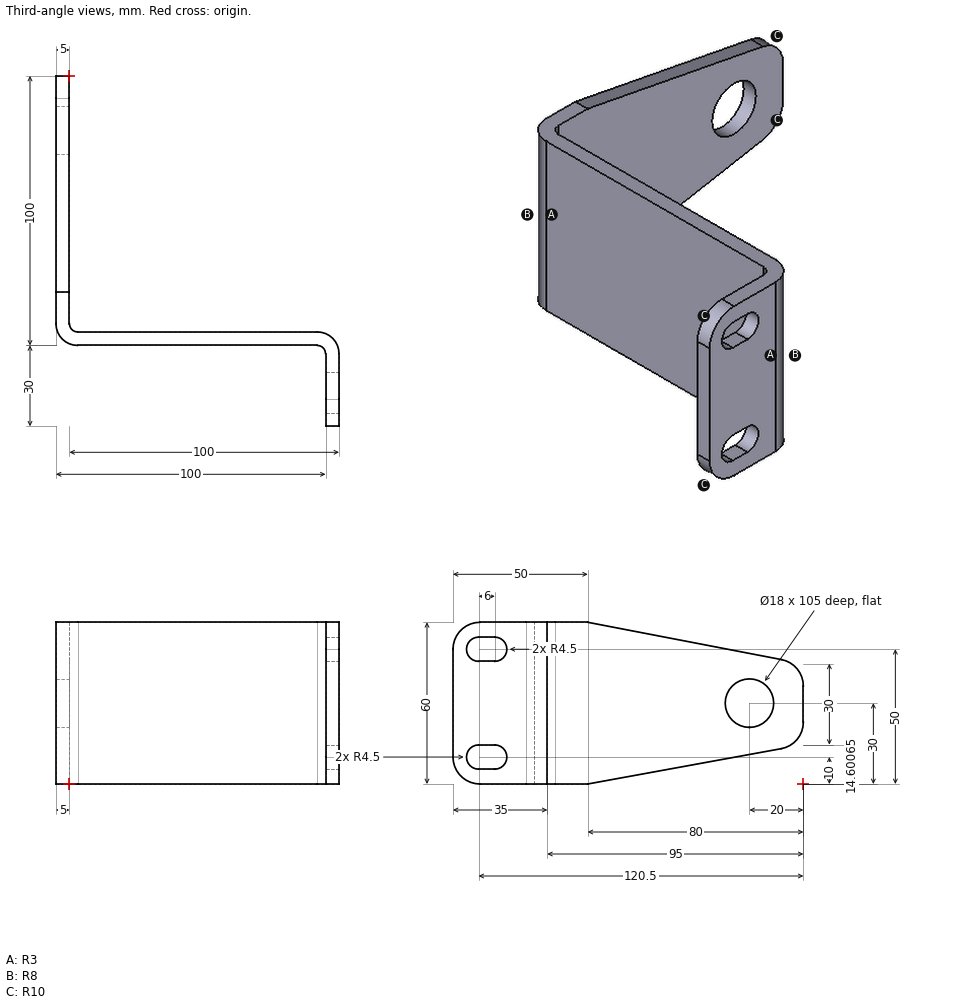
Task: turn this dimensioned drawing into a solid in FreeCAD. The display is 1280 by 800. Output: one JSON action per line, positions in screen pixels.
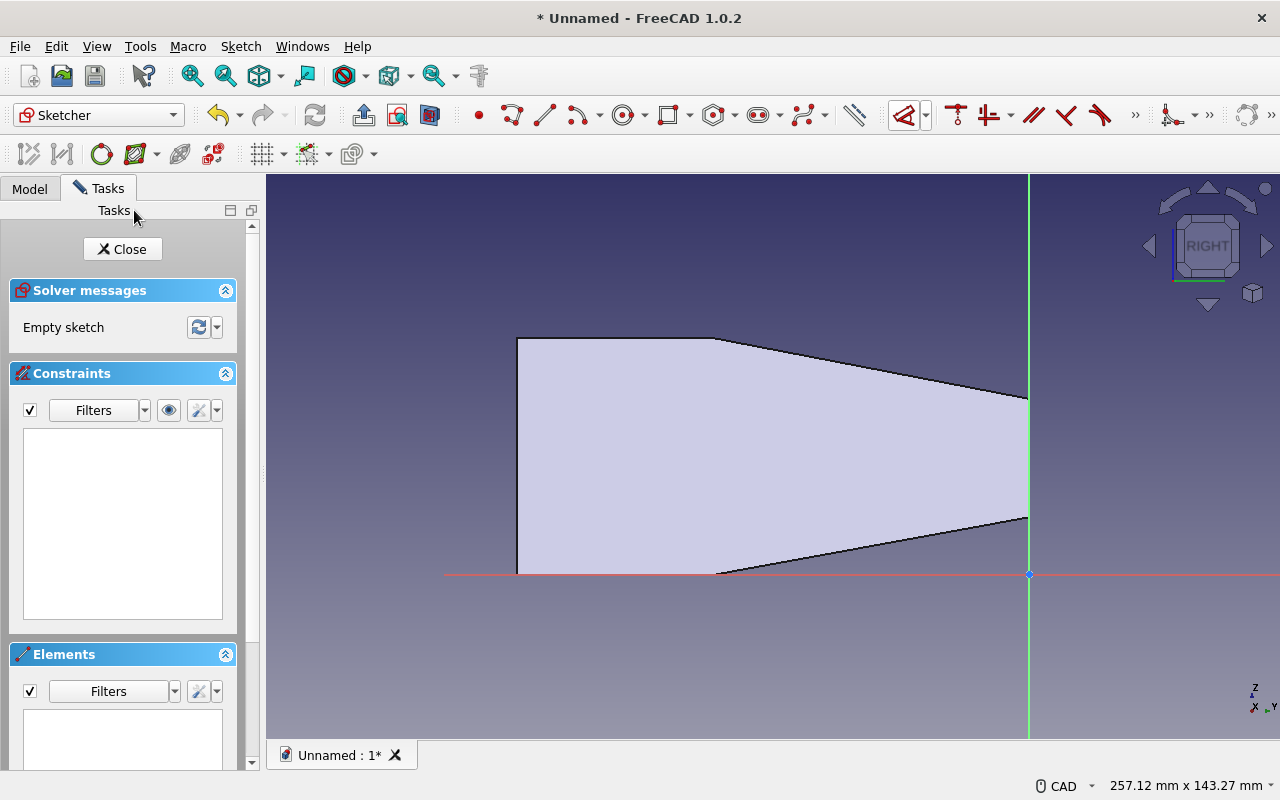
{"action": "left_click", "coordinate": [668, 116]}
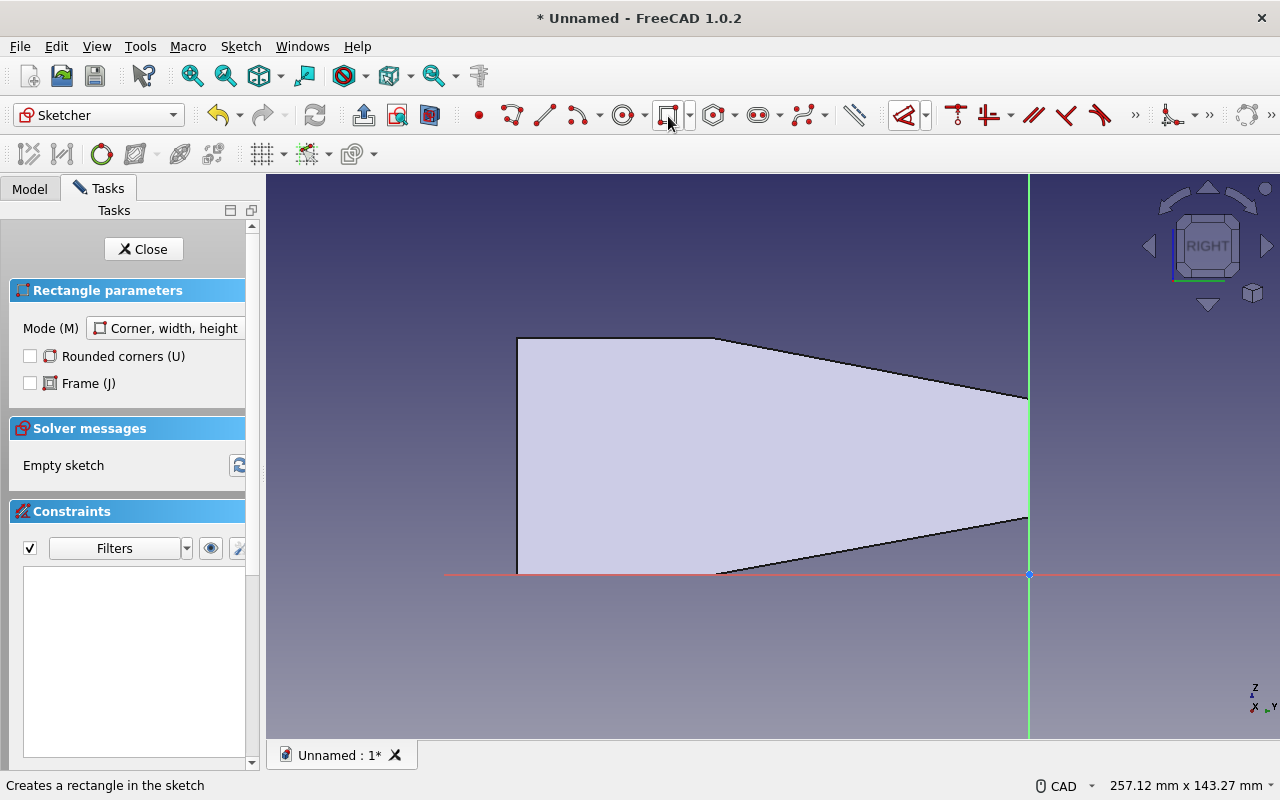
{"action": "left_click", "coordinate": [517, 338]}
{"action": "left_click", "coordinate": [655, 575]}
{"action": "key", "text": "Escape"}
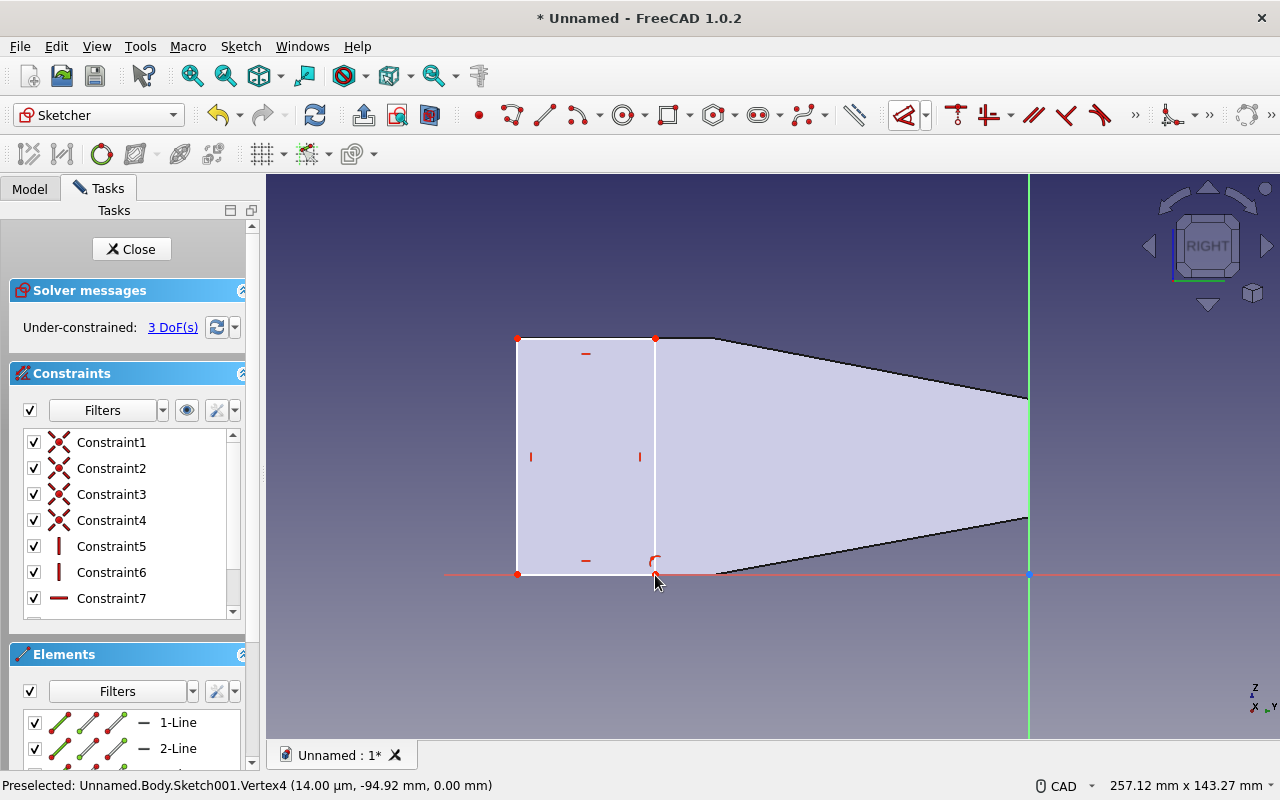
{"action": "left_click", "coordinate": [517, 410]}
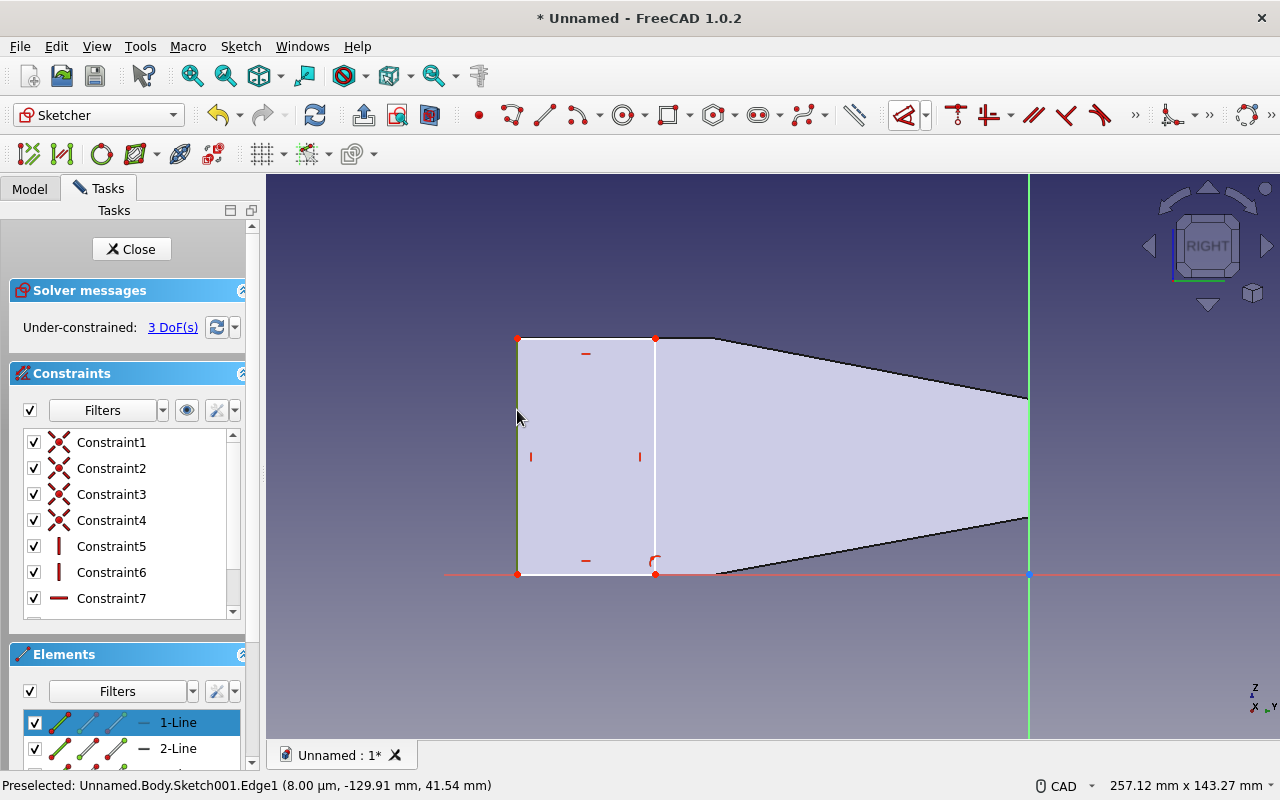
{"action": "key", "text": "i"}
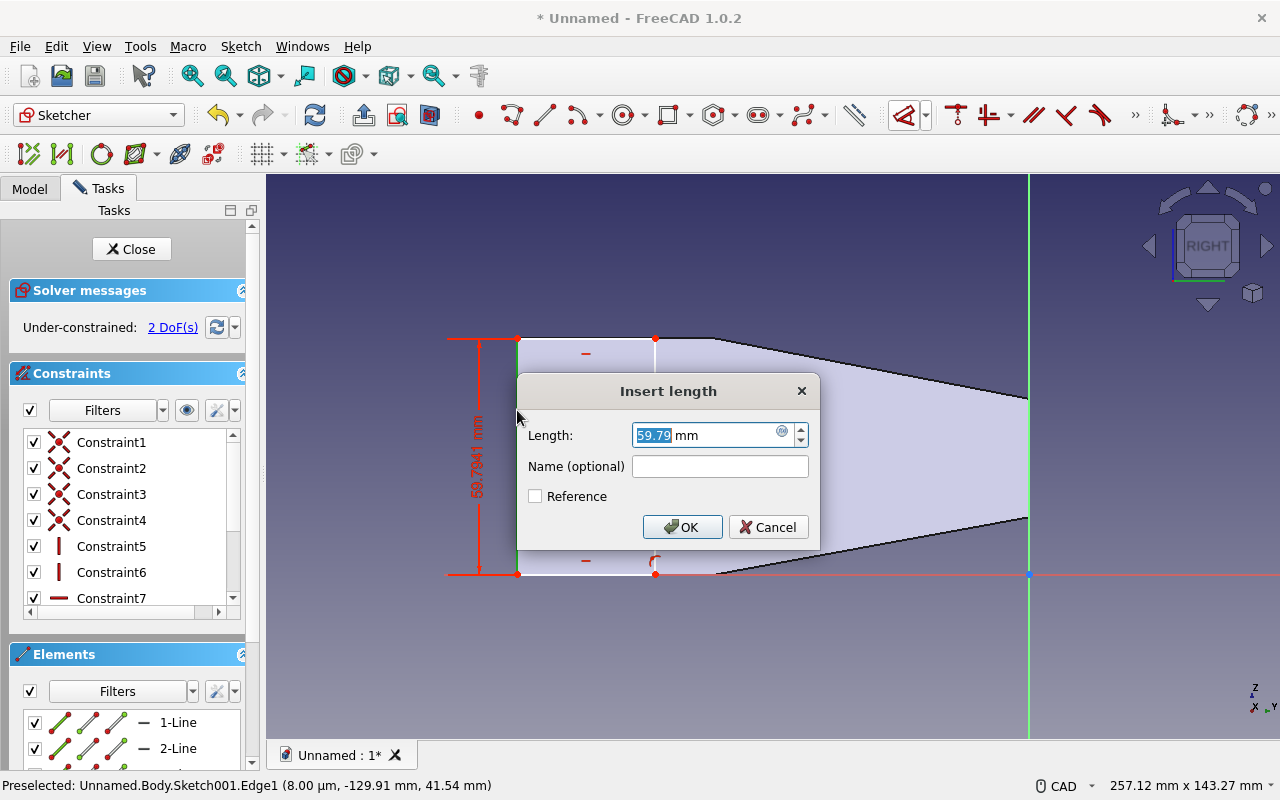
{"action": "type", "text": "60"}
{"action": "key", "text": "Return"}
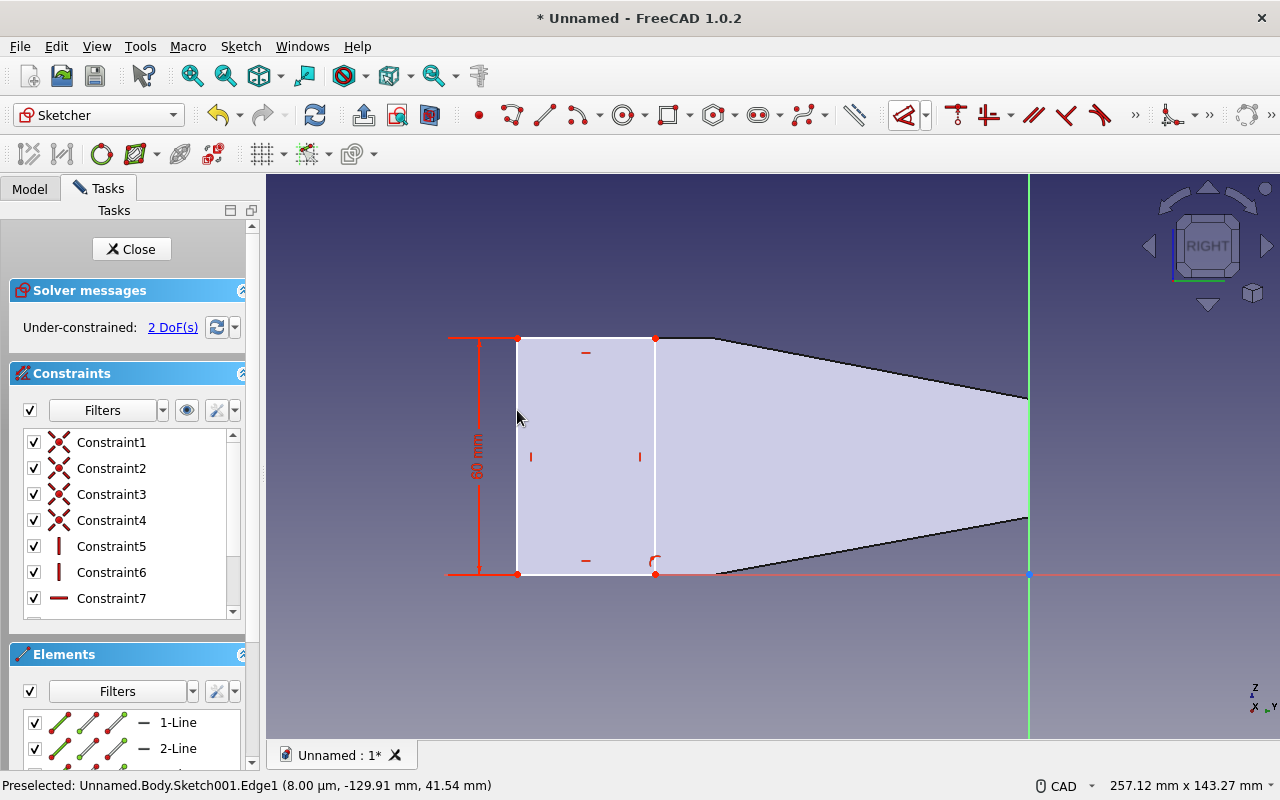
{"action": "left_click", "coordinate": [558, 575]}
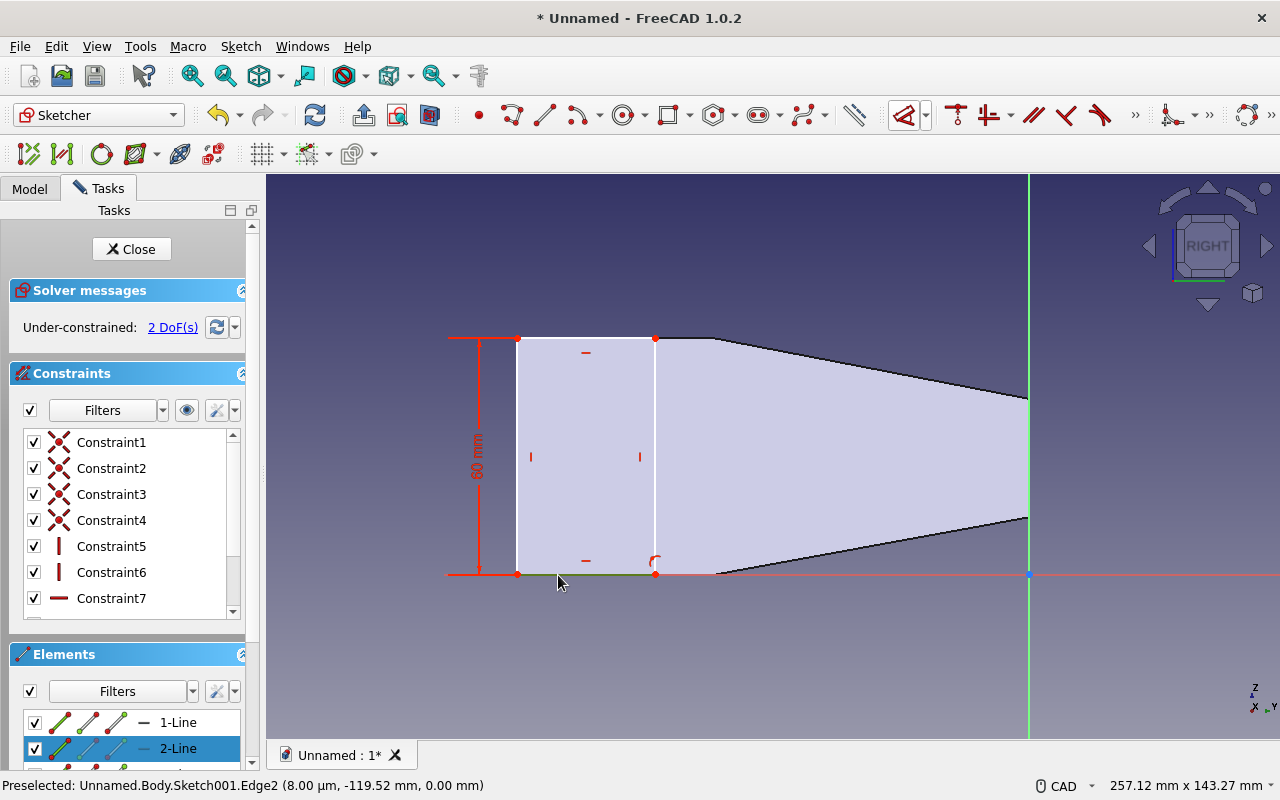
{"action": "key", "text": "l"}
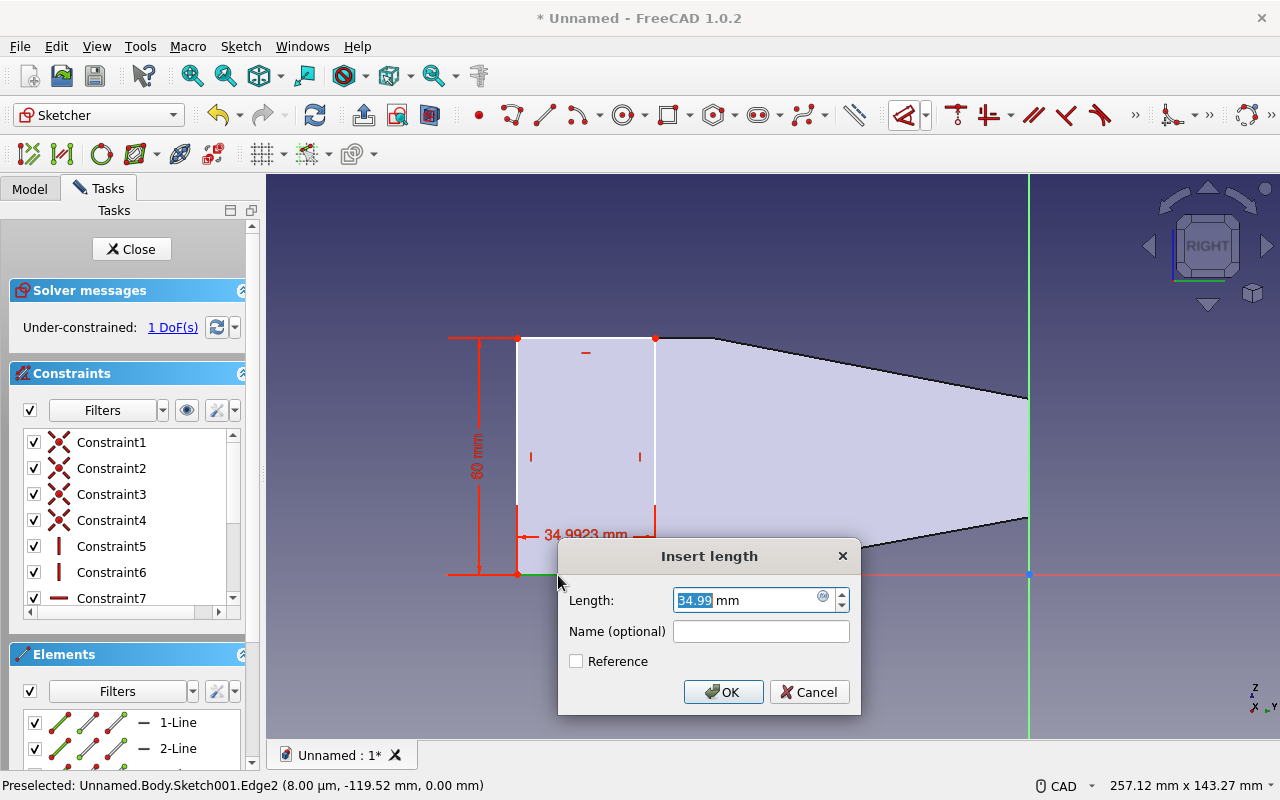
{"action": "type", "text": "35"}
{"action": "key", "text": "Return"}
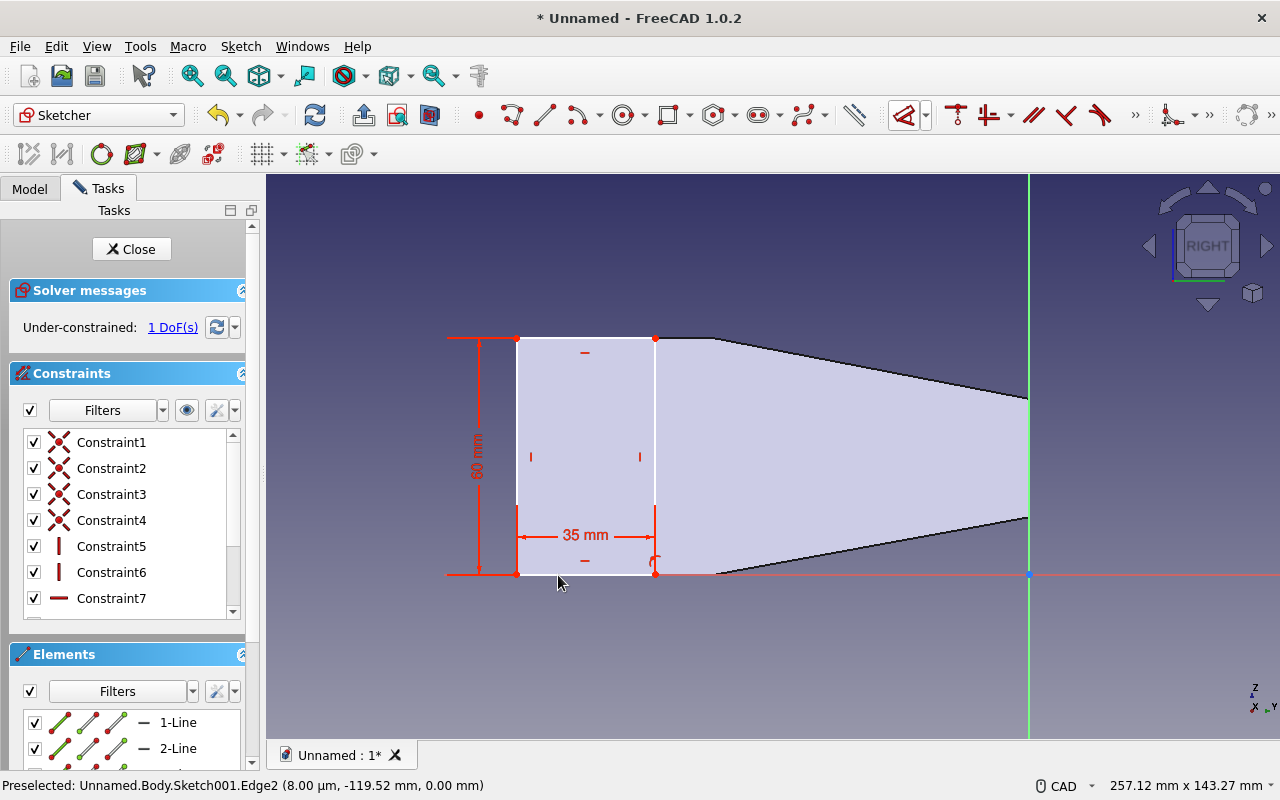
{"action": "left_click", "coordinate": [655, 575]}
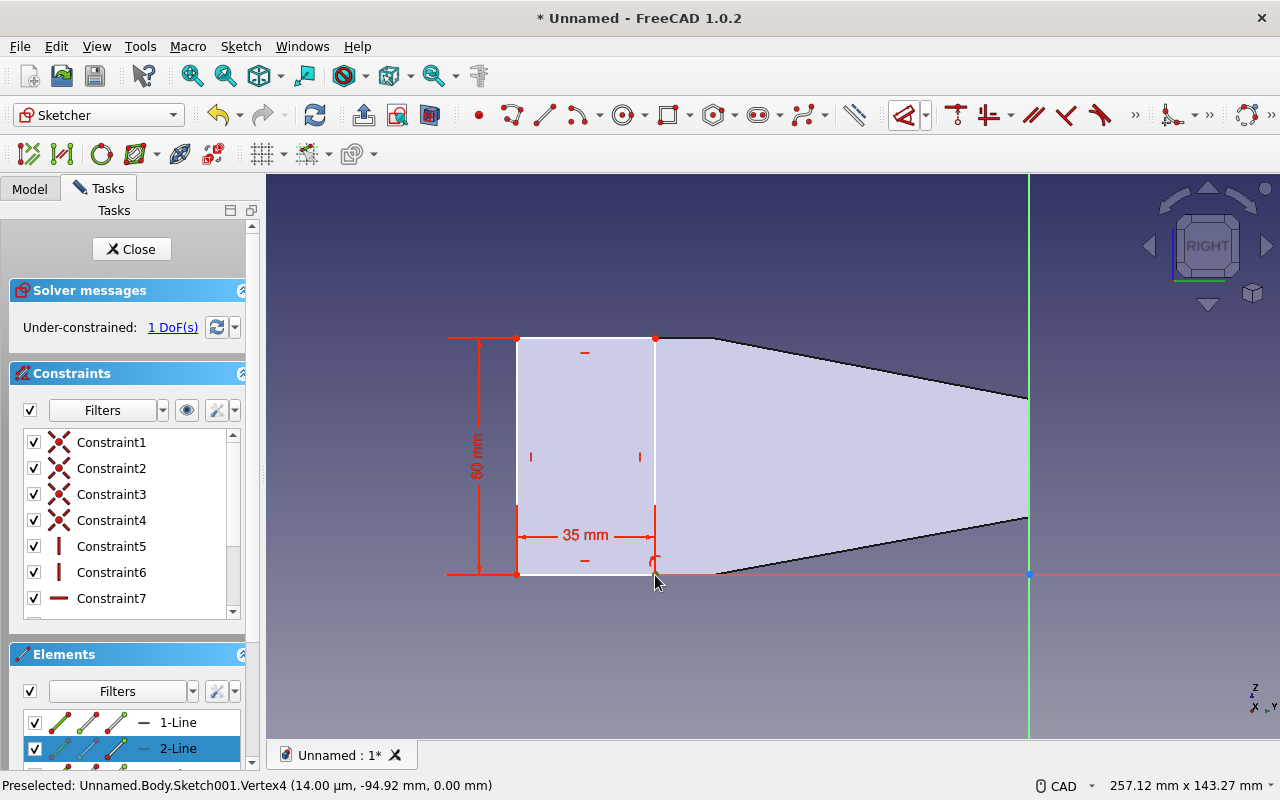
{"action": "key", "text": "l"}